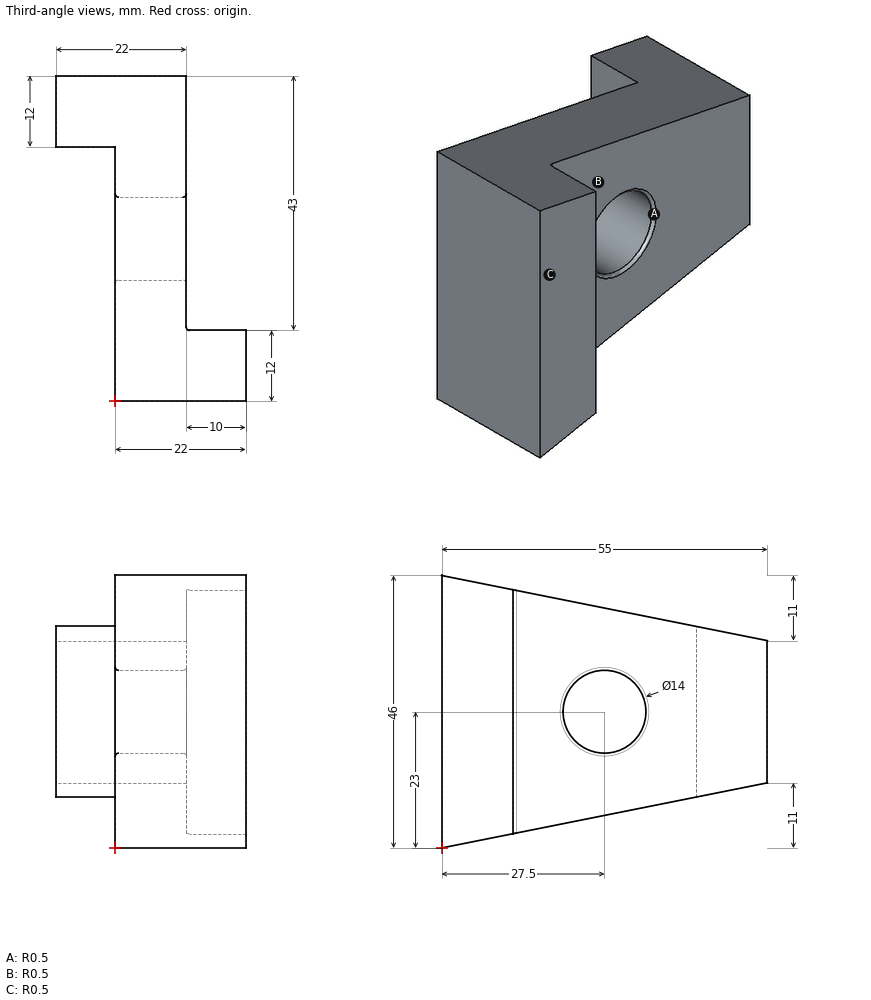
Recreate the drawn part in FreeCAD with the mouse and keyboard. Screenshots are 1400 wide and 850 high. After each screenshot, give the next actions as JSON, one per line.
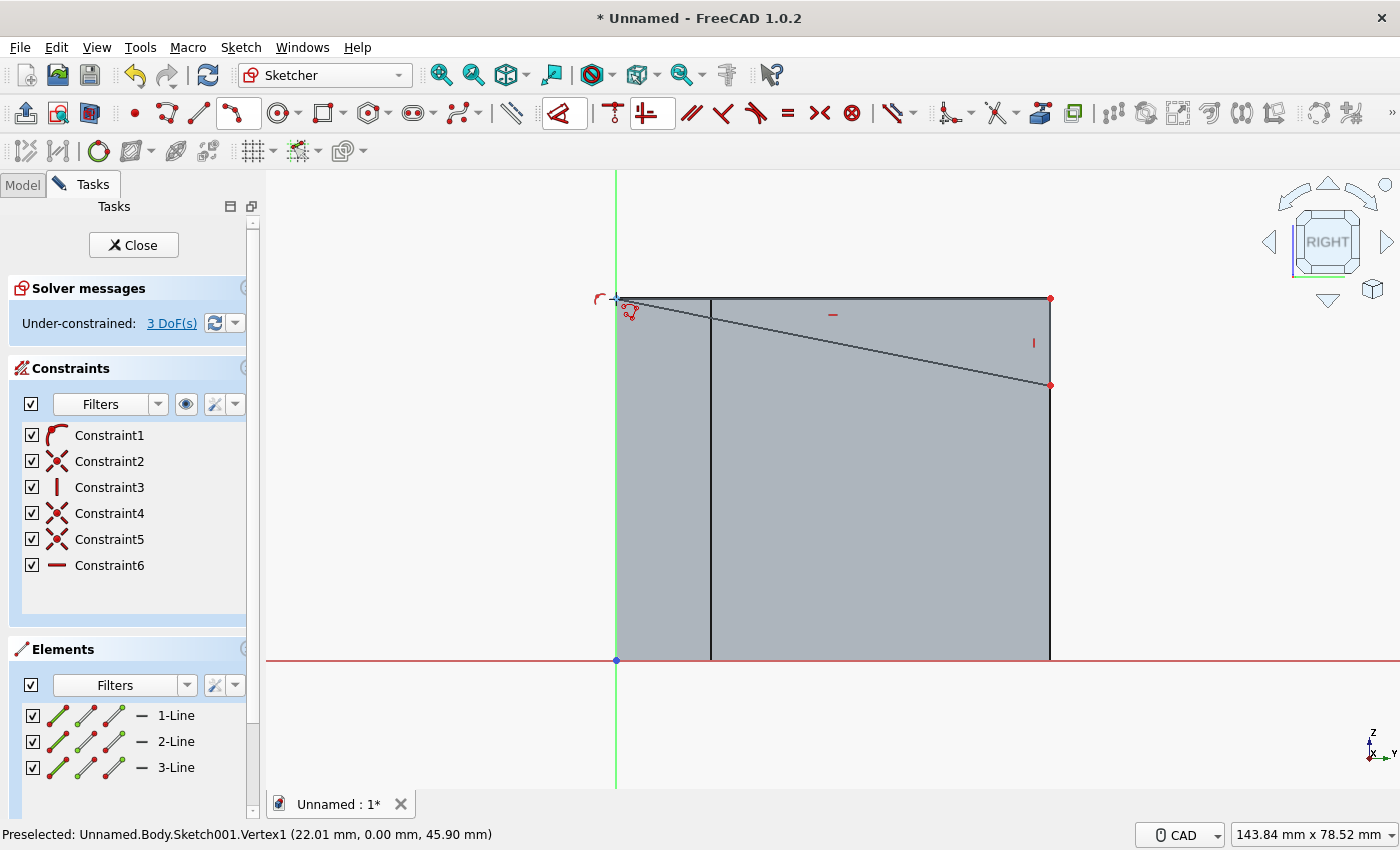
{"action": "left_click", "coordinate": [616, 661]}
{"action": "left_click", "coordinate": [1050, 652]}
{"action": "left_click", "coordinate": [1050, 574]}
{"action": "left_click", "coordinate": [616, 661]}
{"action": "key", "text": "Escape"}
{"action": "key", "text": "Escape"}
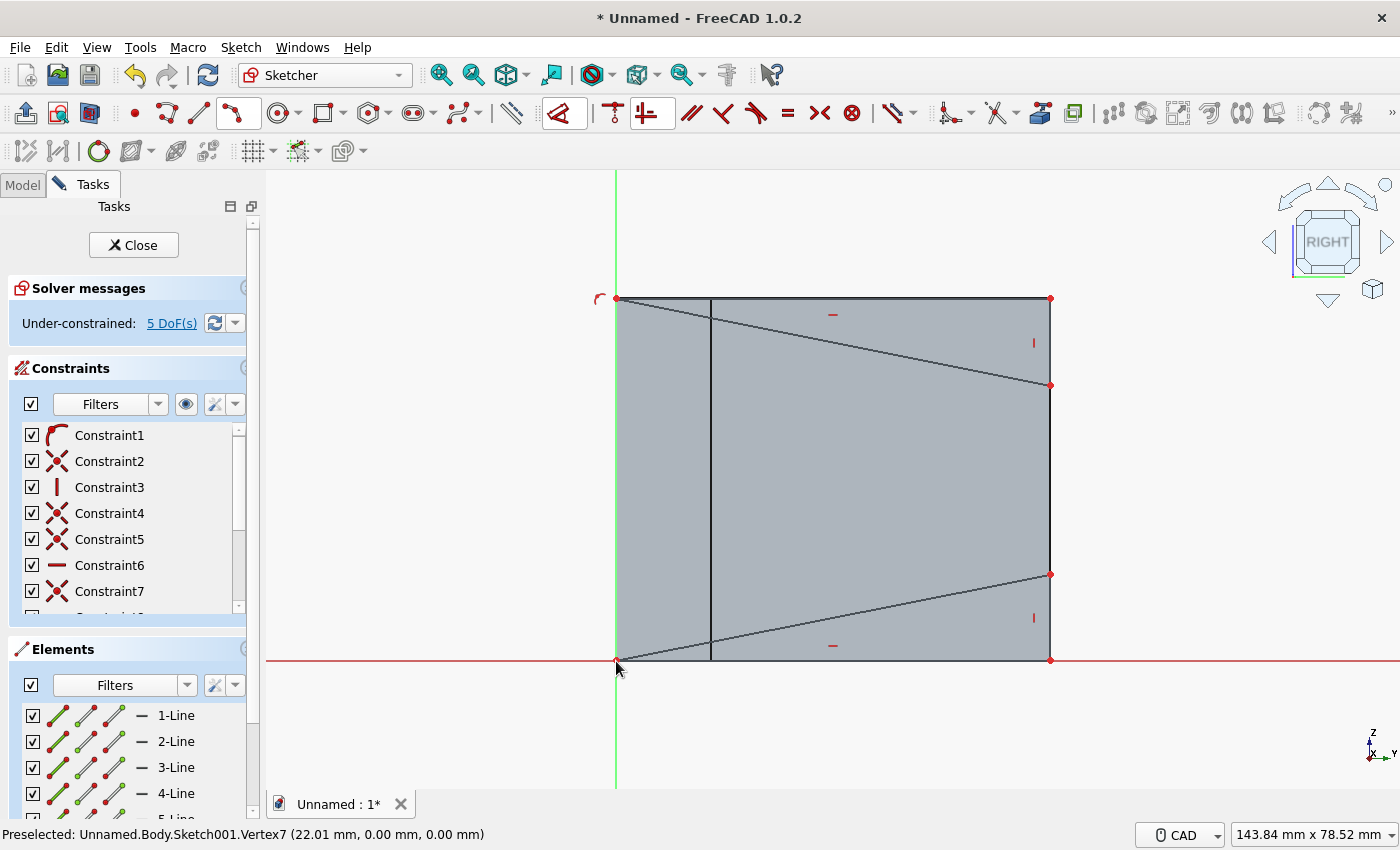
{"action": "left_click", "coordinate": [1050, 360]}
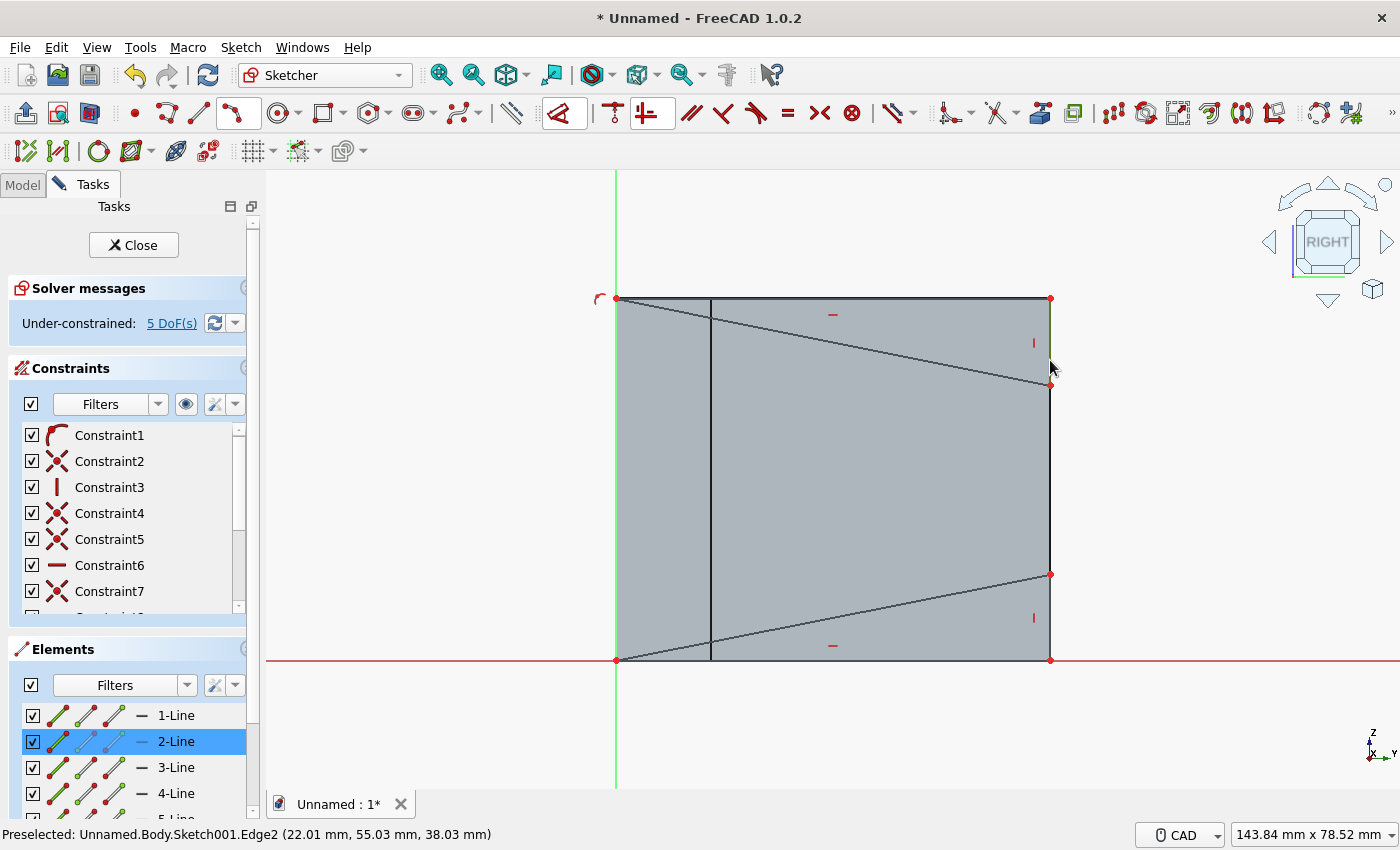
{"action": "key", "text": "i"}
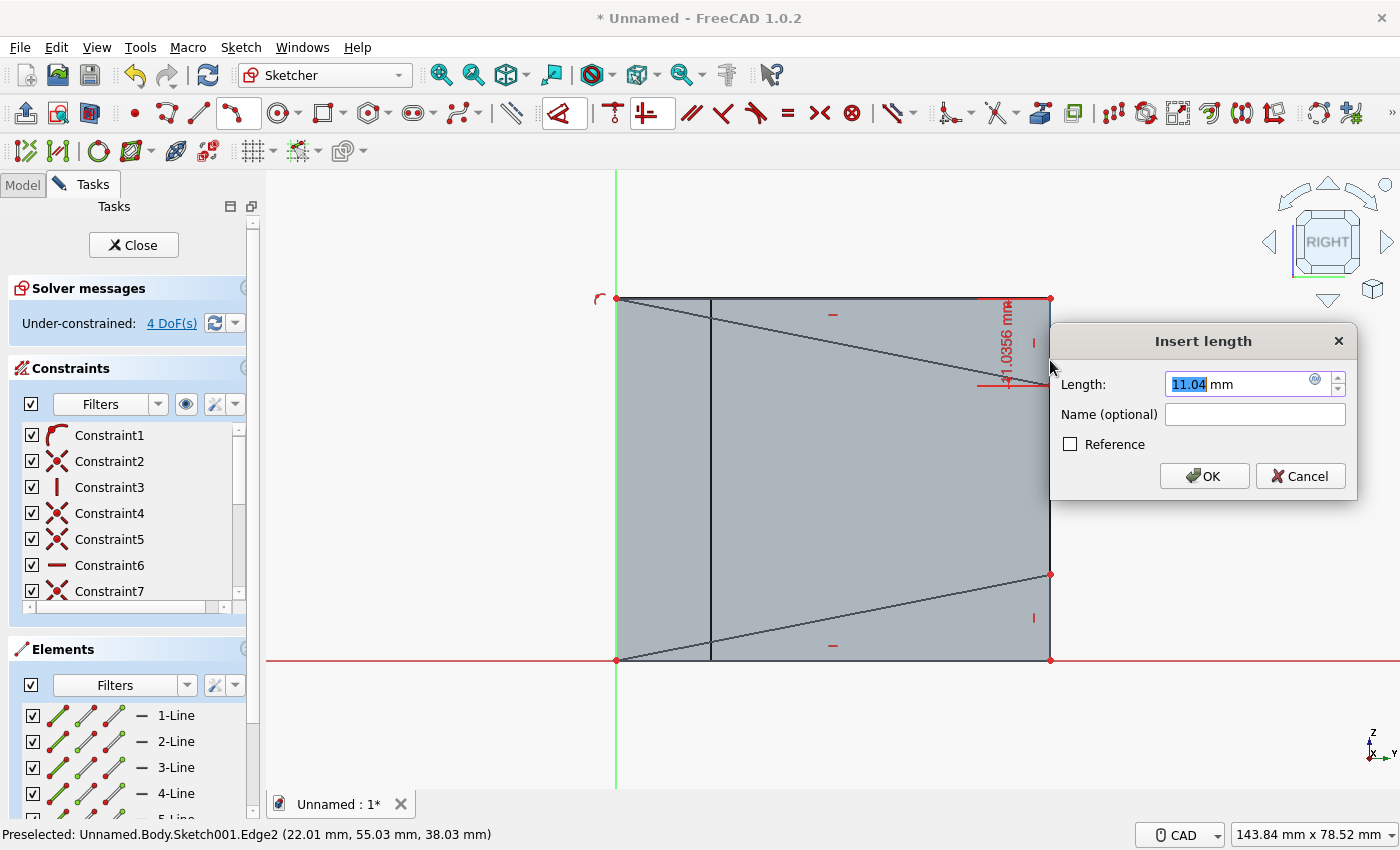
{"action": "type", "text": "11"}
{"action": "key", "text": "Return"}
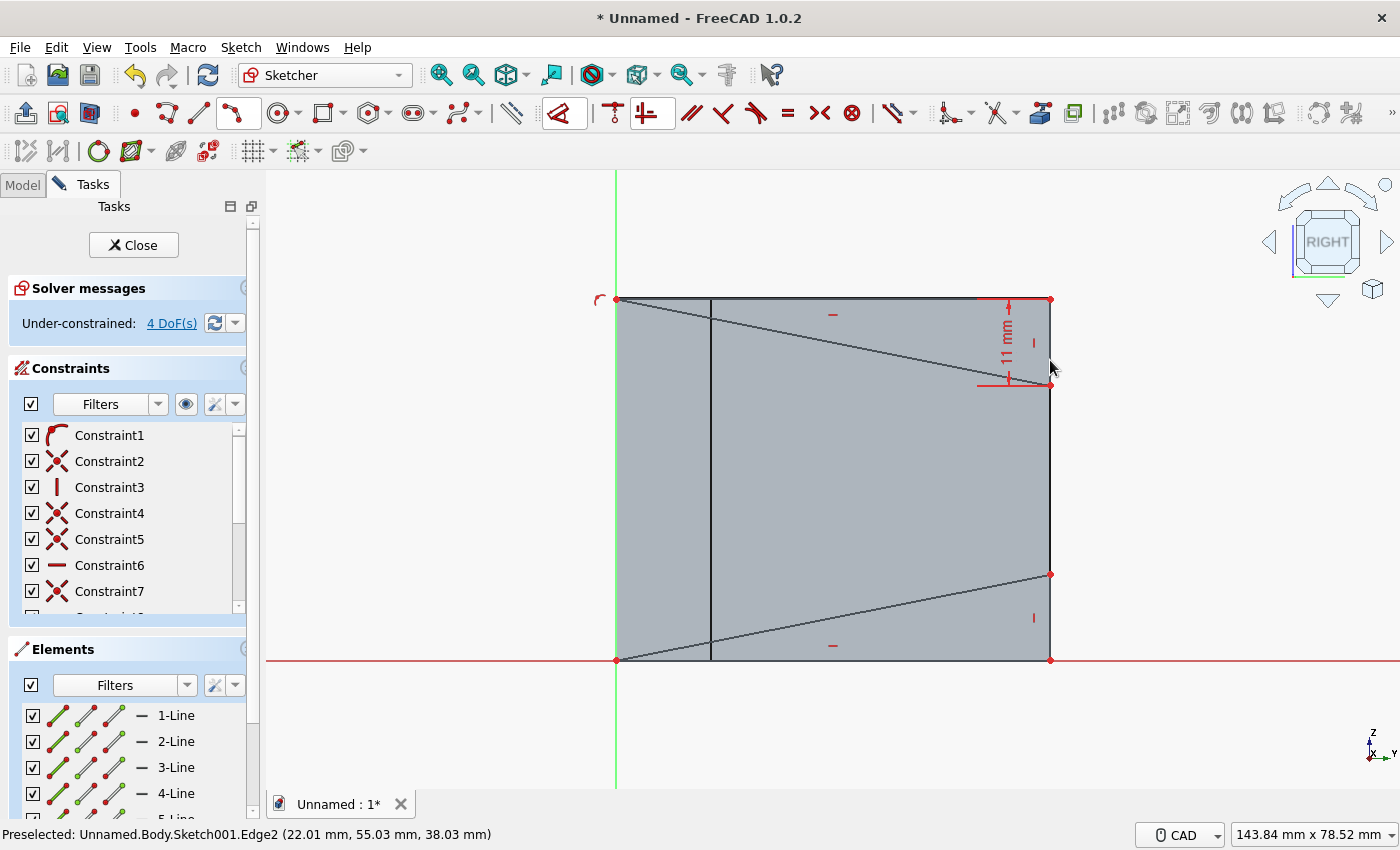
{"action": "left_click", "coordinate": [920, 299]}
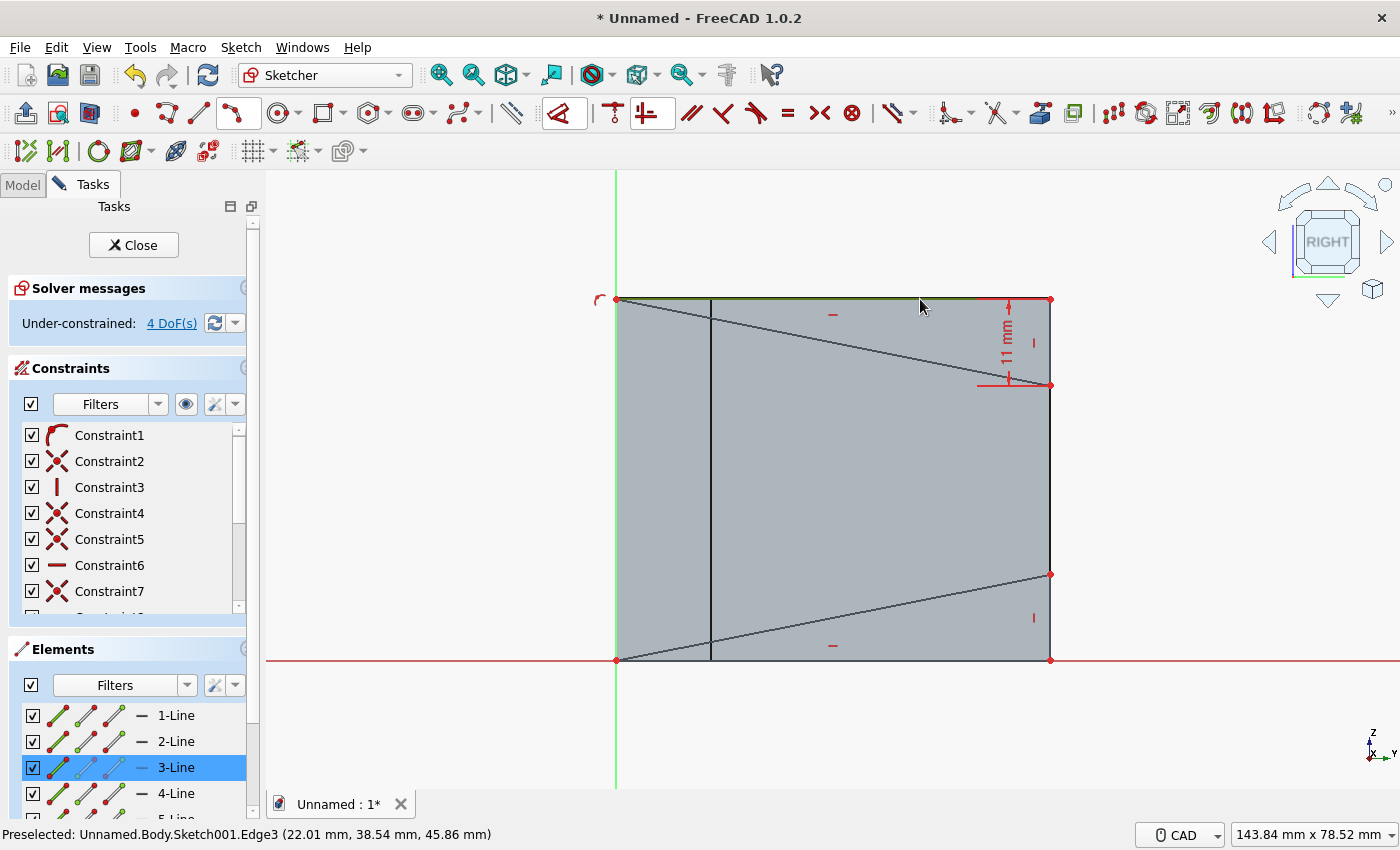
{"action": "key", "text": "l"}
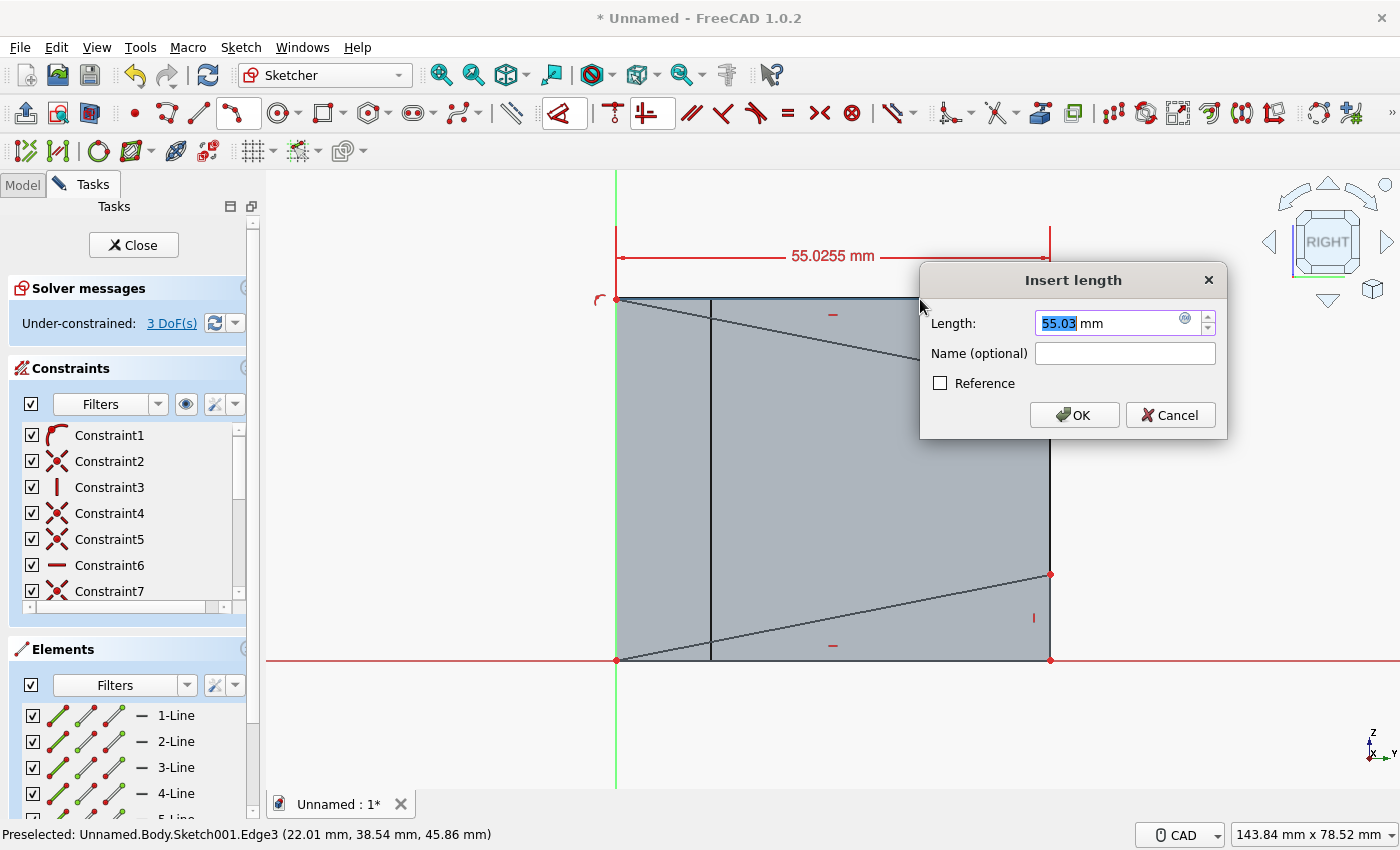
{"action": "type", "text": "55"}
{"action": "key", "text": "Return"}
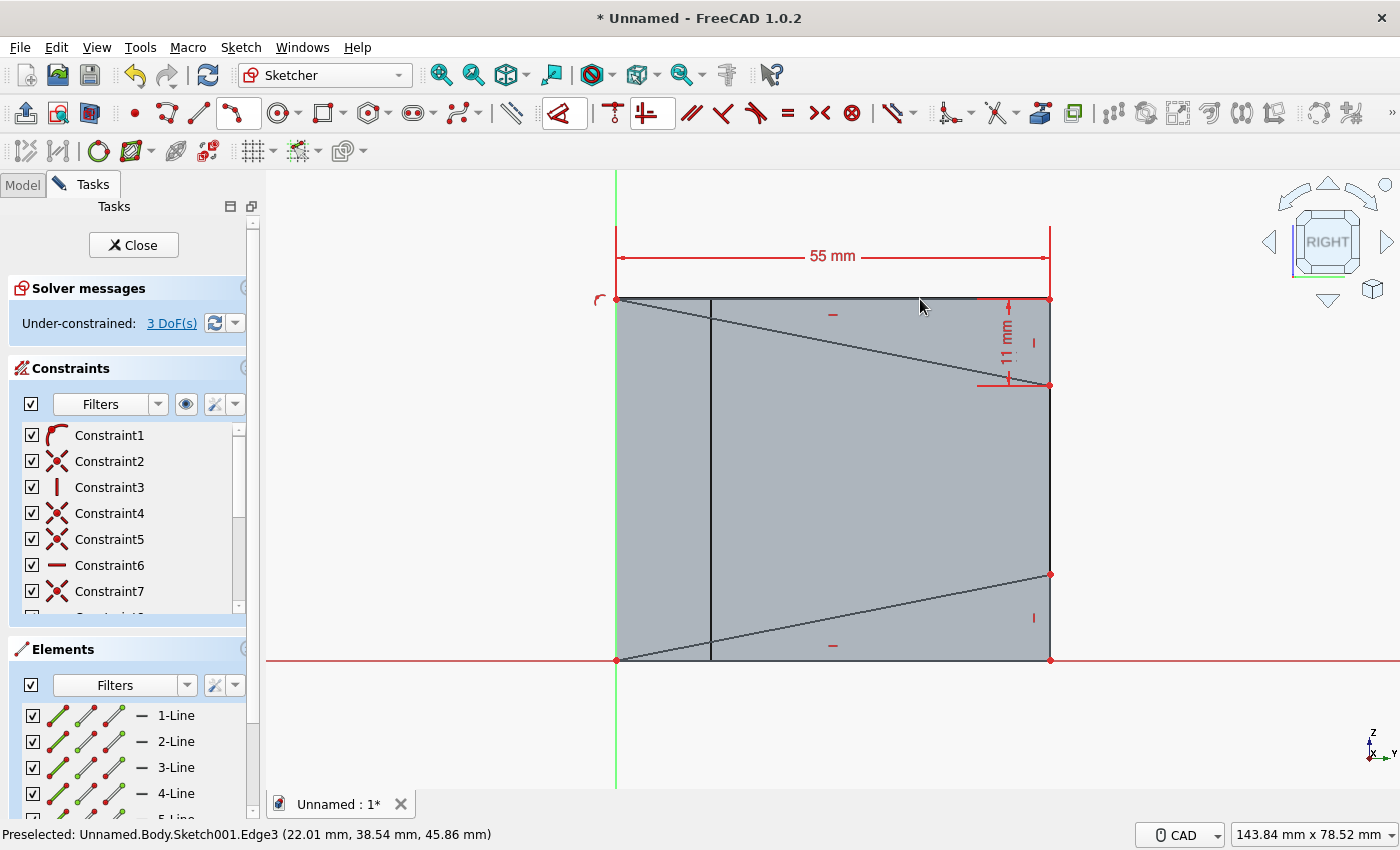
{"action": "left_click", "coordinate": [746, 661]}